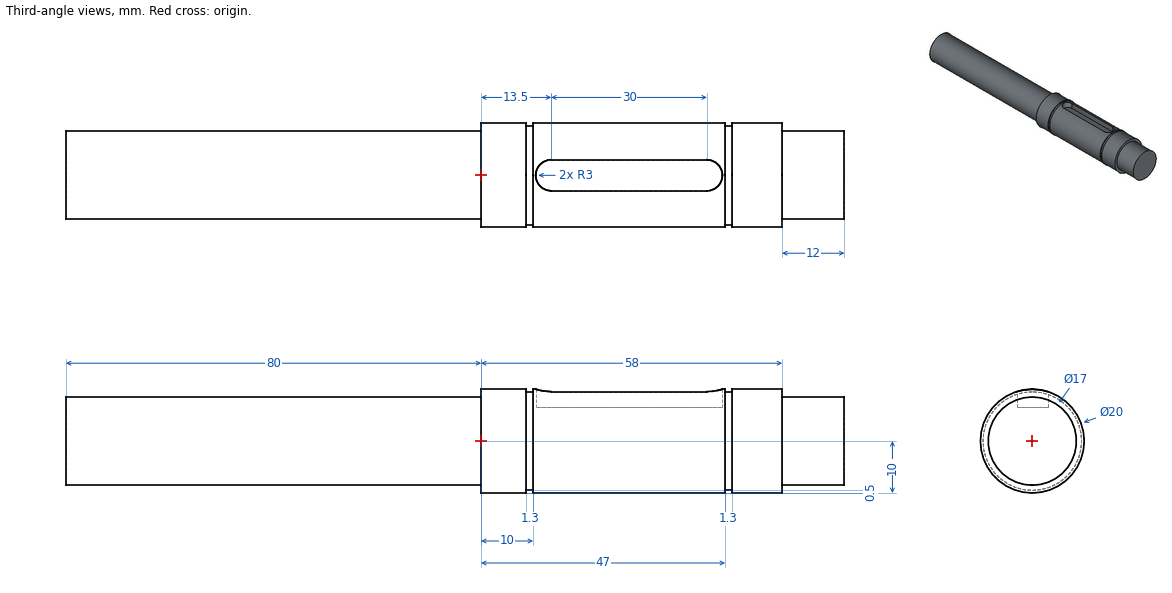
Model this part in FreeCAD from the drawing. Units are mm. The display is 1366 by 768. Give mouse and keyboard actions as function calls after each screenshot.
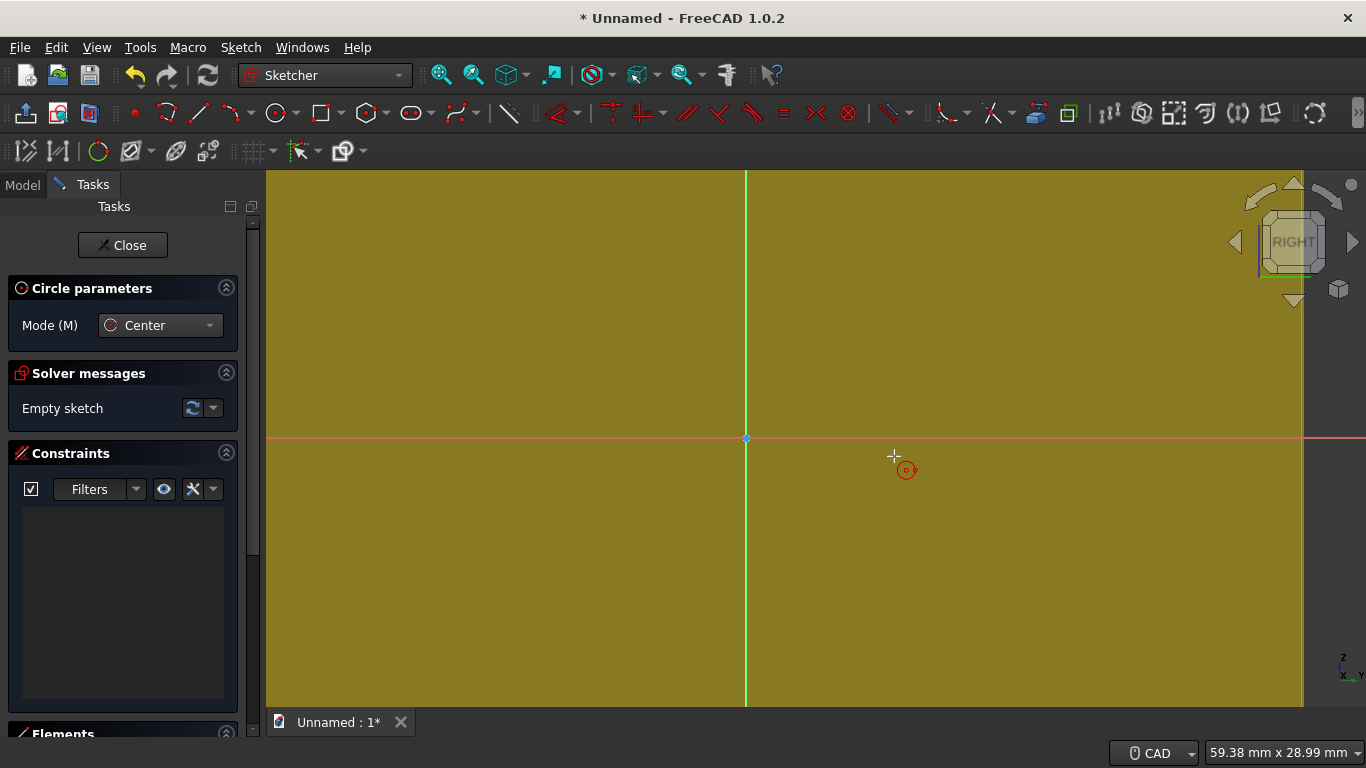
click(746, 438)
click(858, 327)
key(Escape)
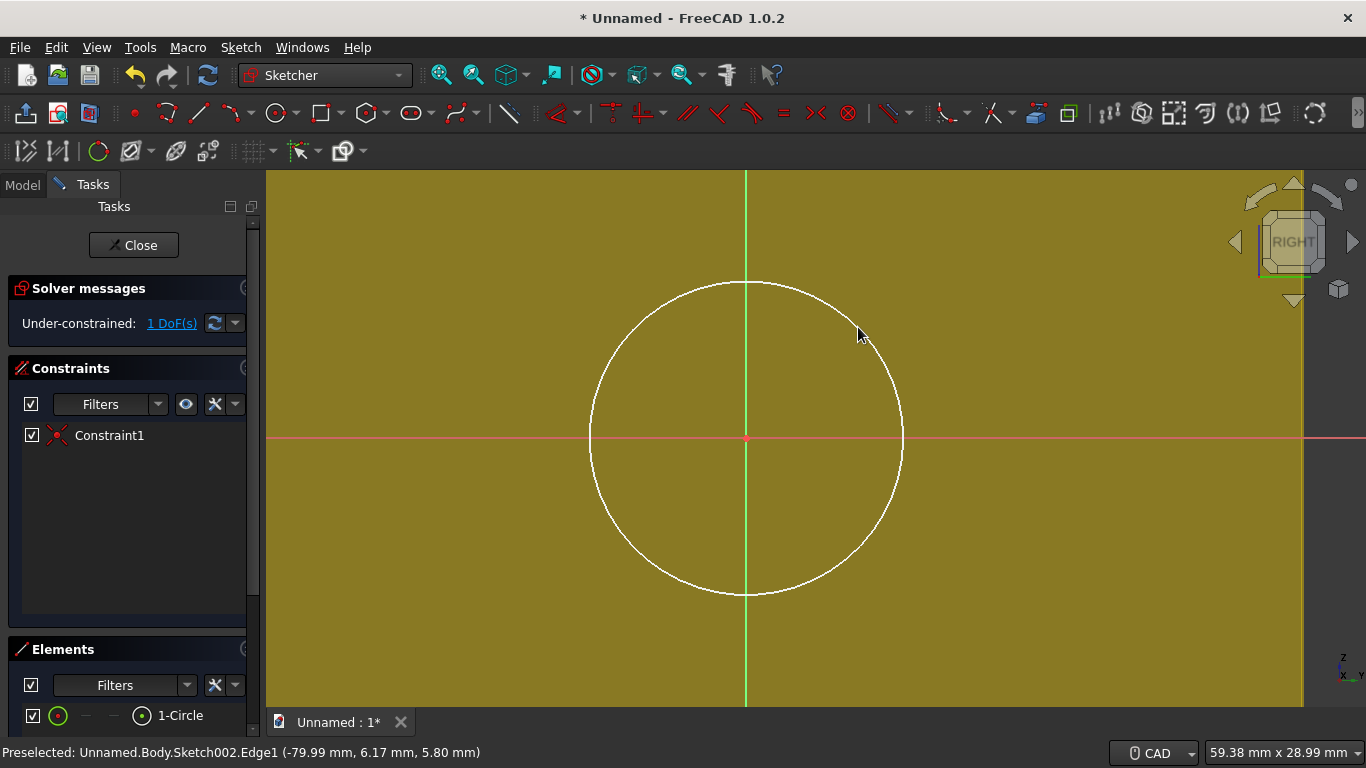
click(556, 114)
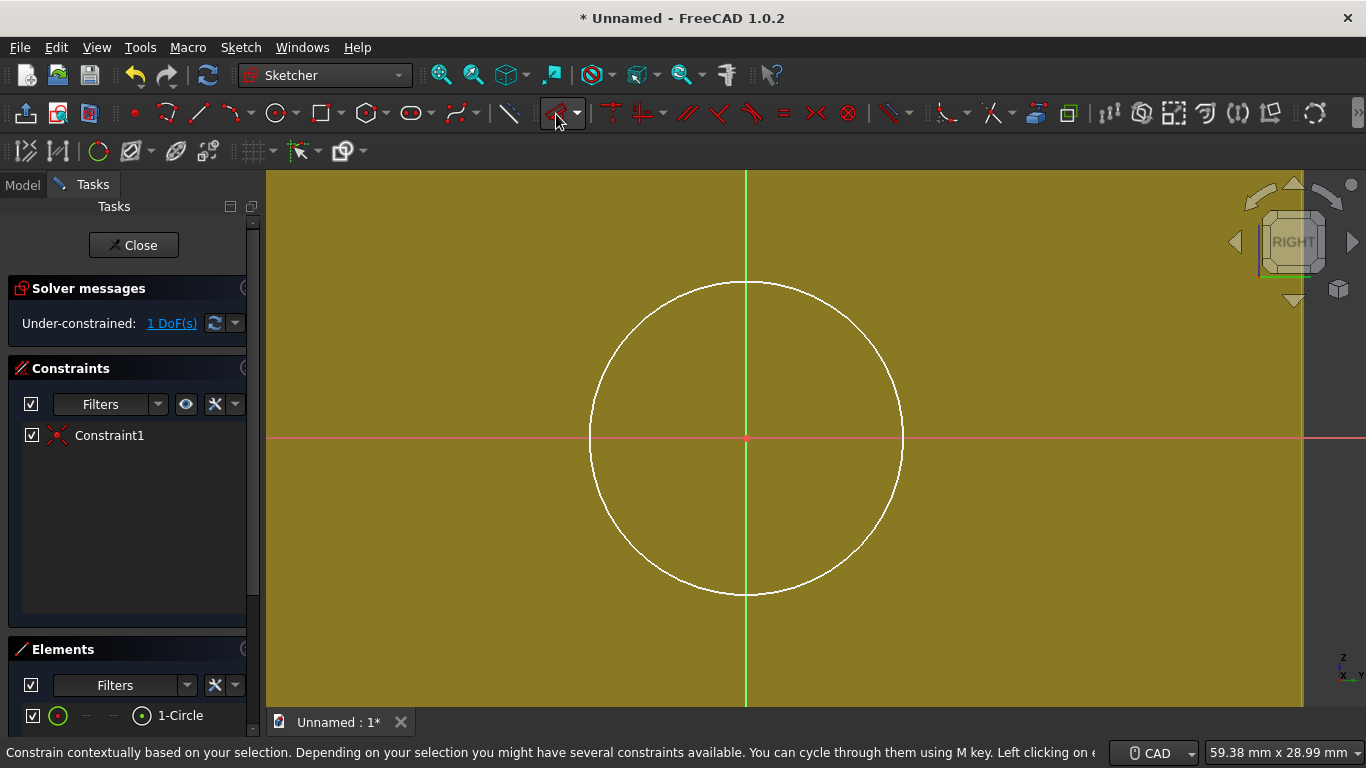
click(857, 327)
click(880, 304)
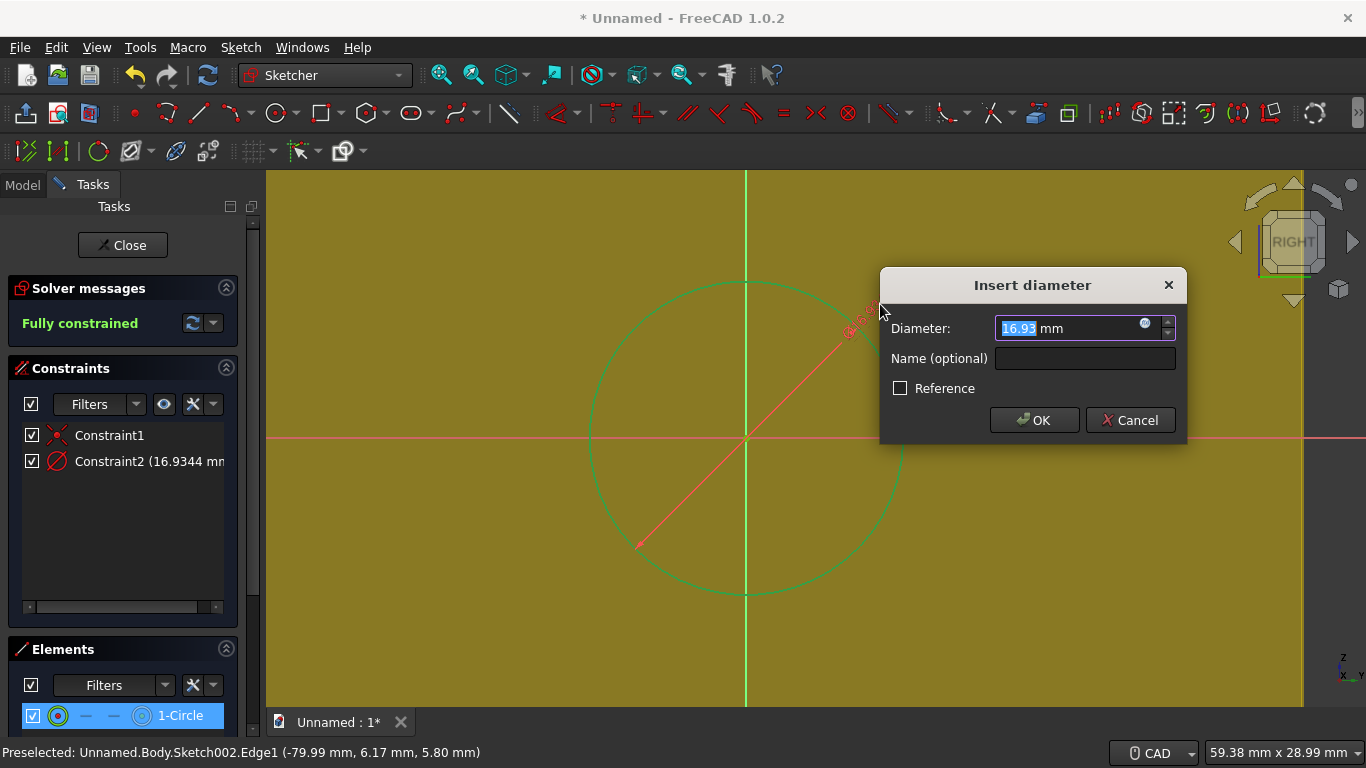
text(17)
key(Return)
key(Escape)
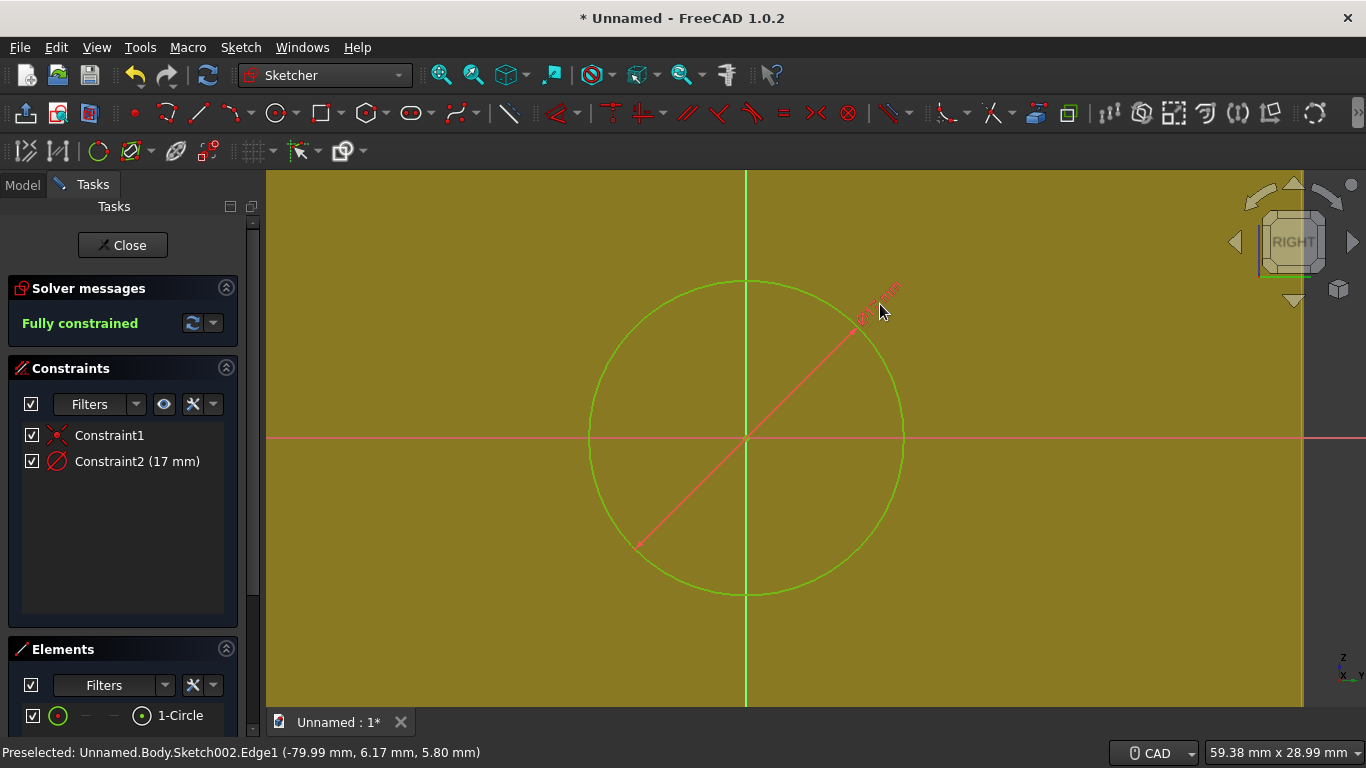
click(123, 245)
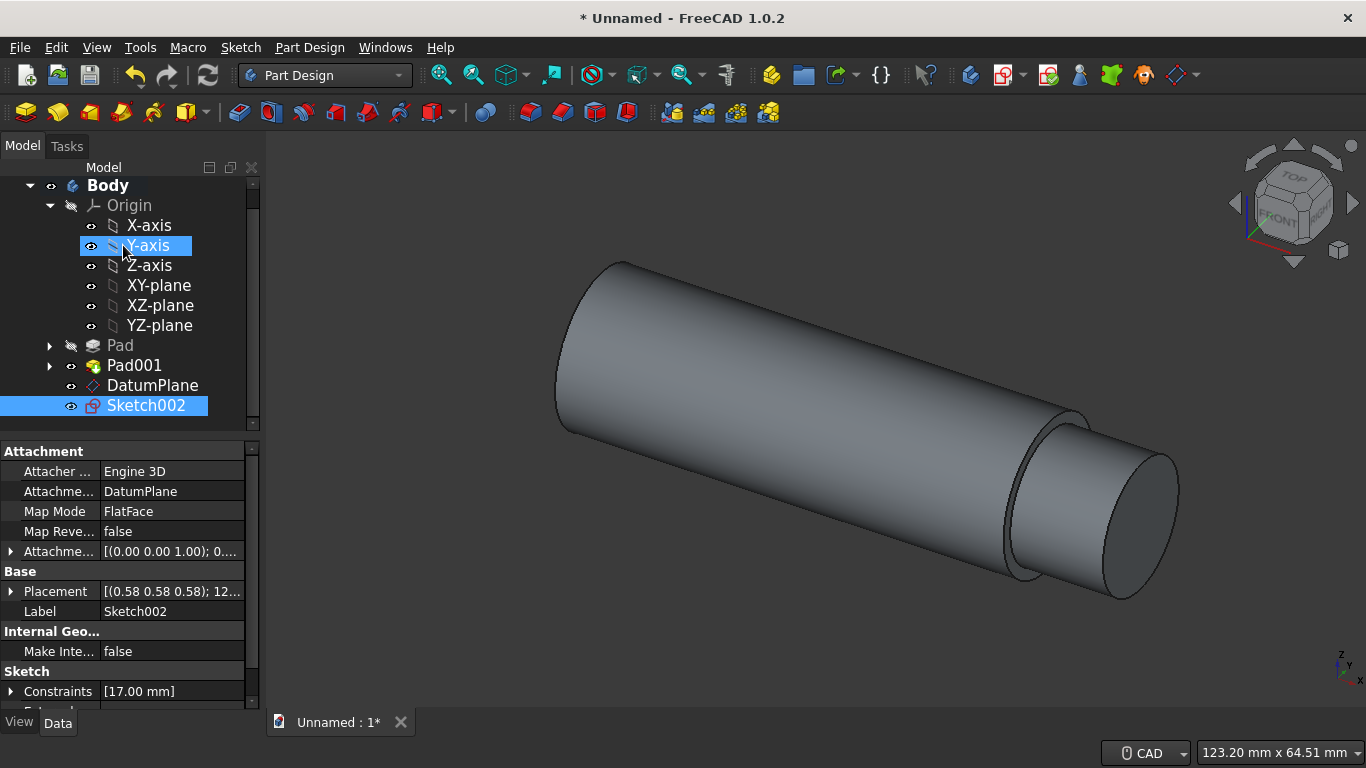
click(26, 112)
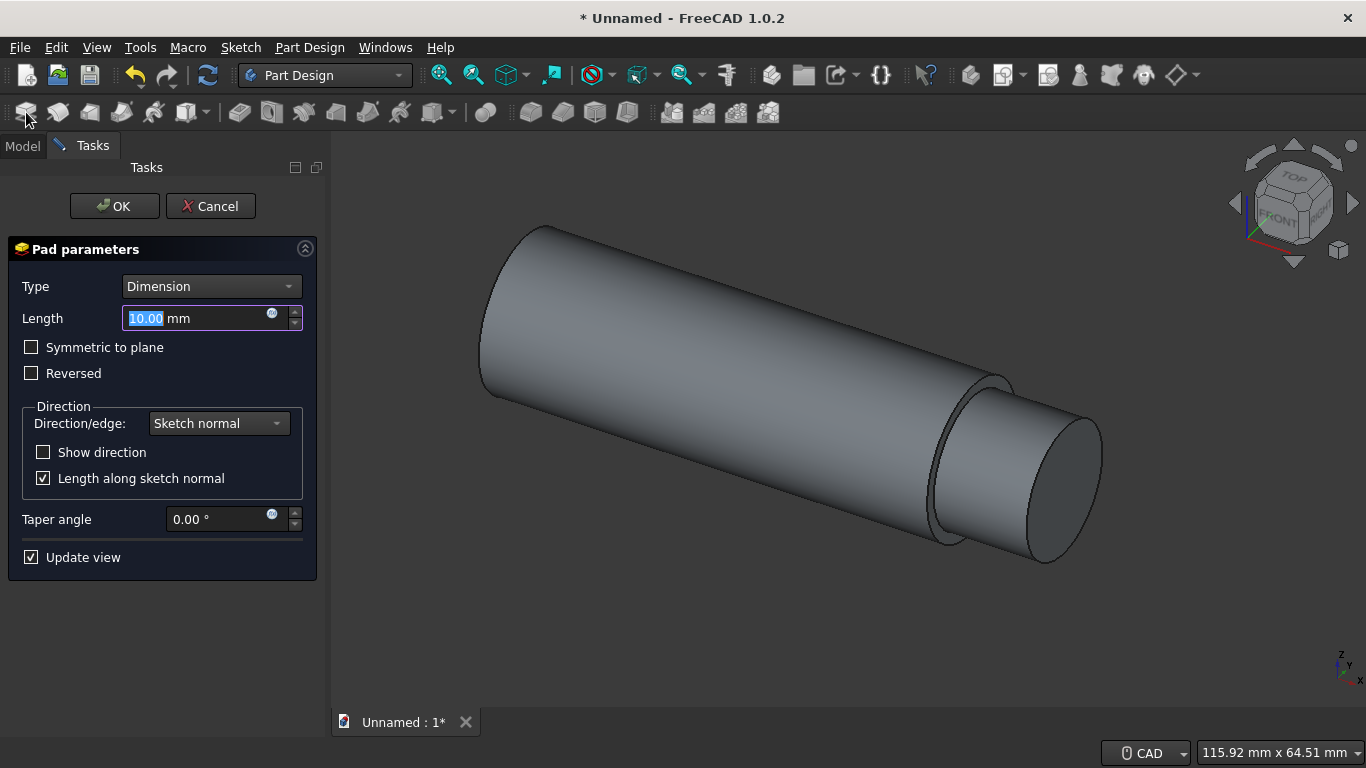
text(80)
key(Tab)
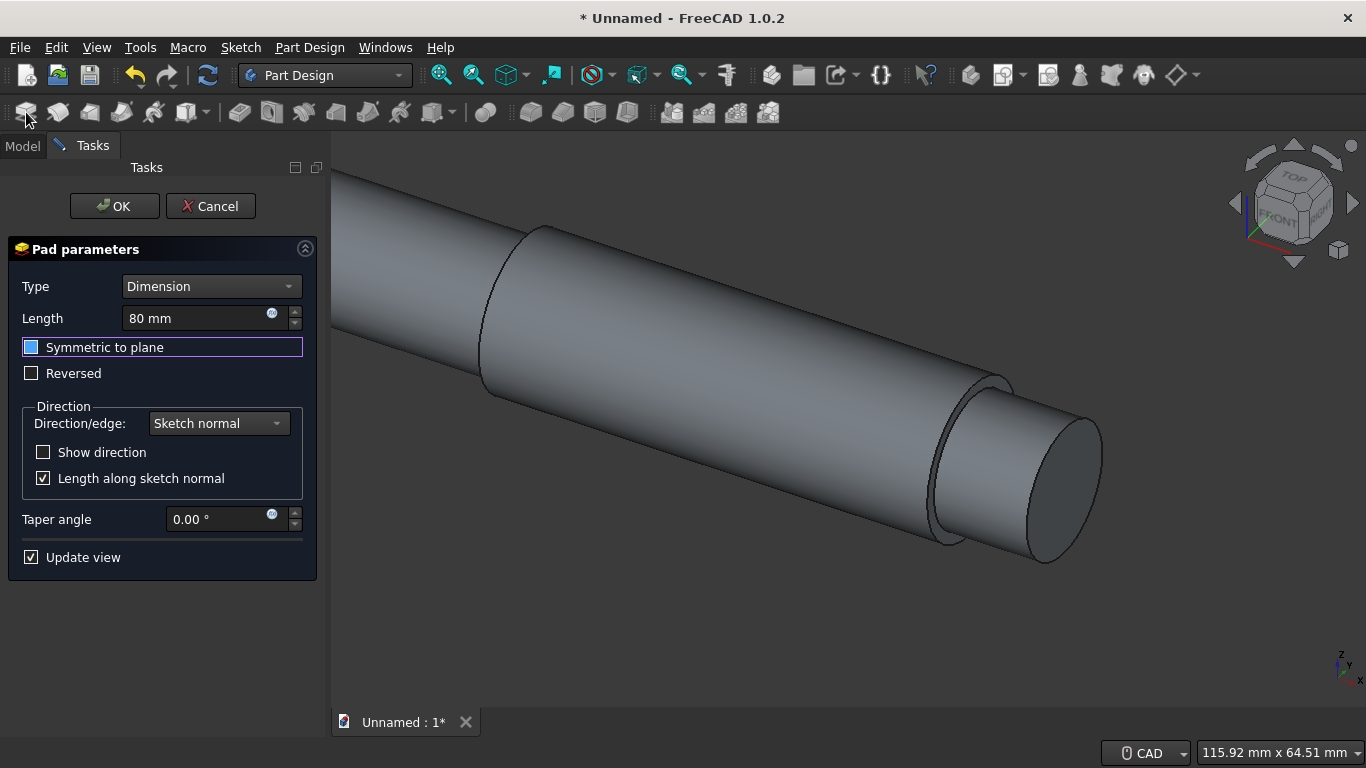
click(115, 206)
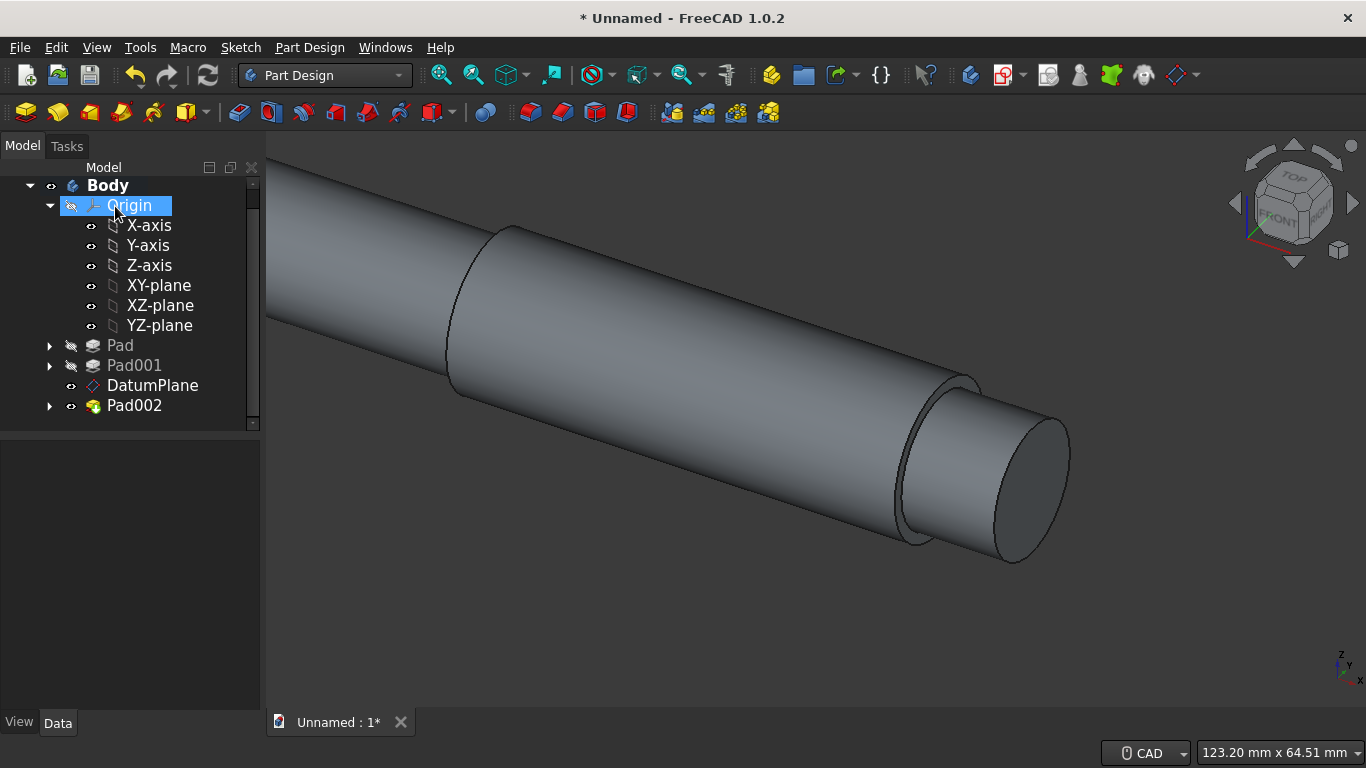
click(116, 386)
key(space)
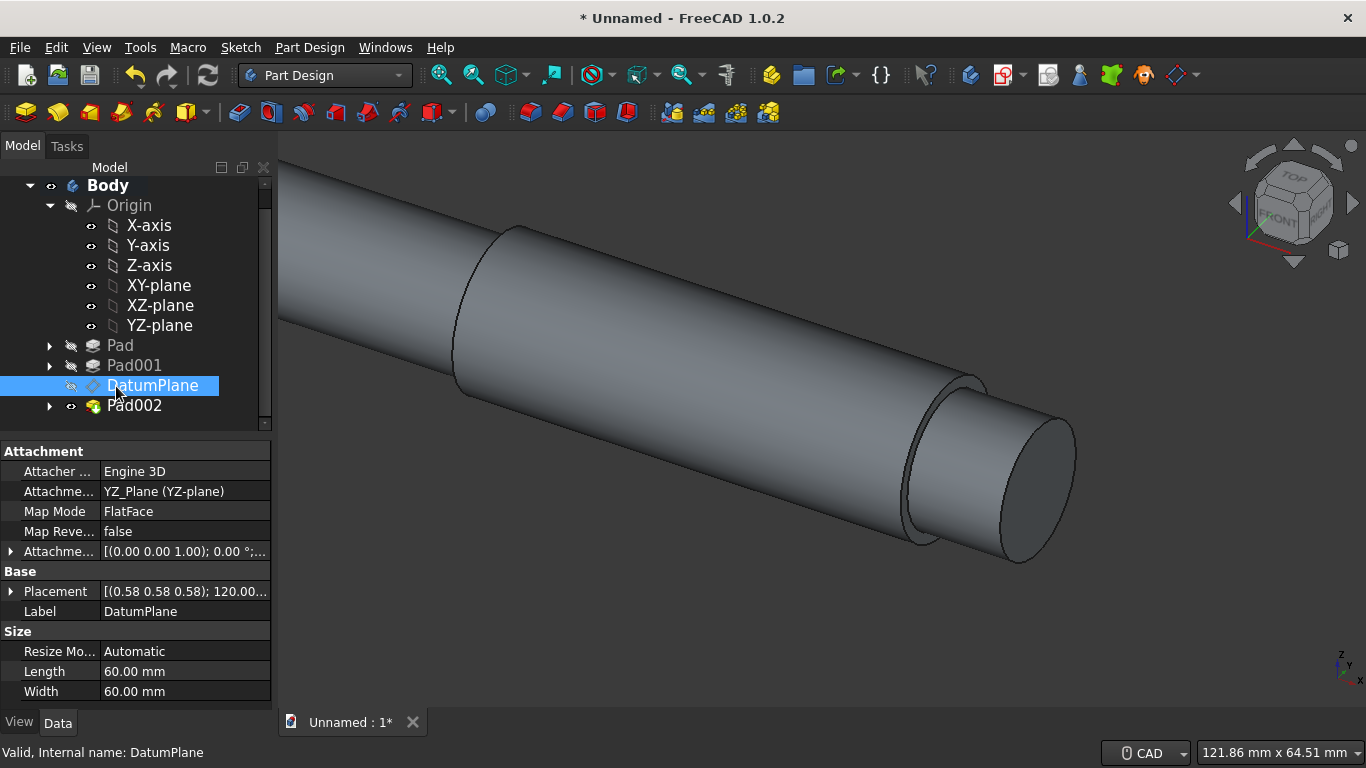
key(v)
key(f)